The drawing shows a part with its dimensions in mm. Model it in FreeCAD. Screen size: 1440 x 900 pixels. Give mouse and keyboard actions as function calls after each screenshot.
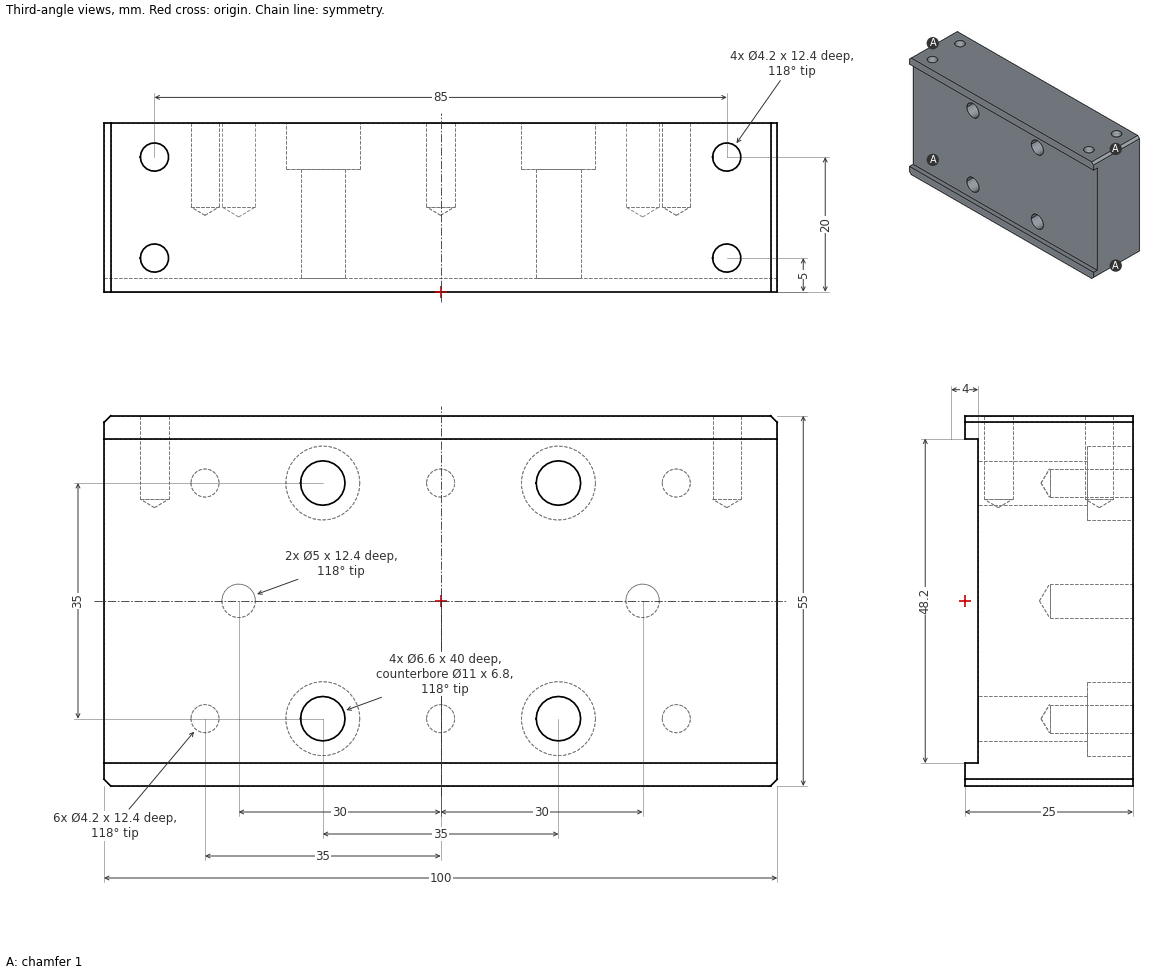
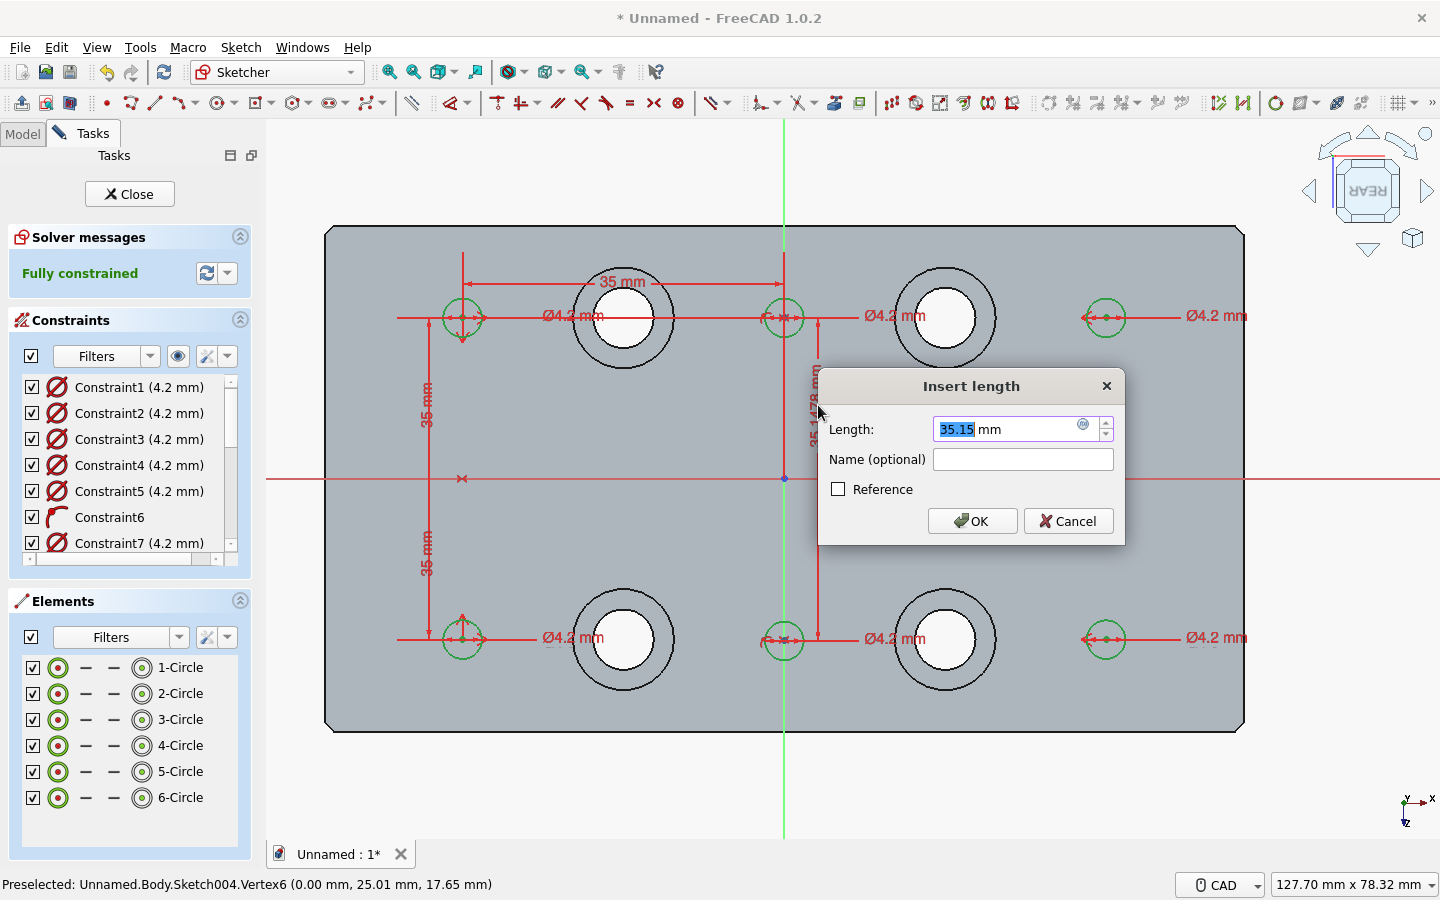
text(35)
key(Return)
key(Escape)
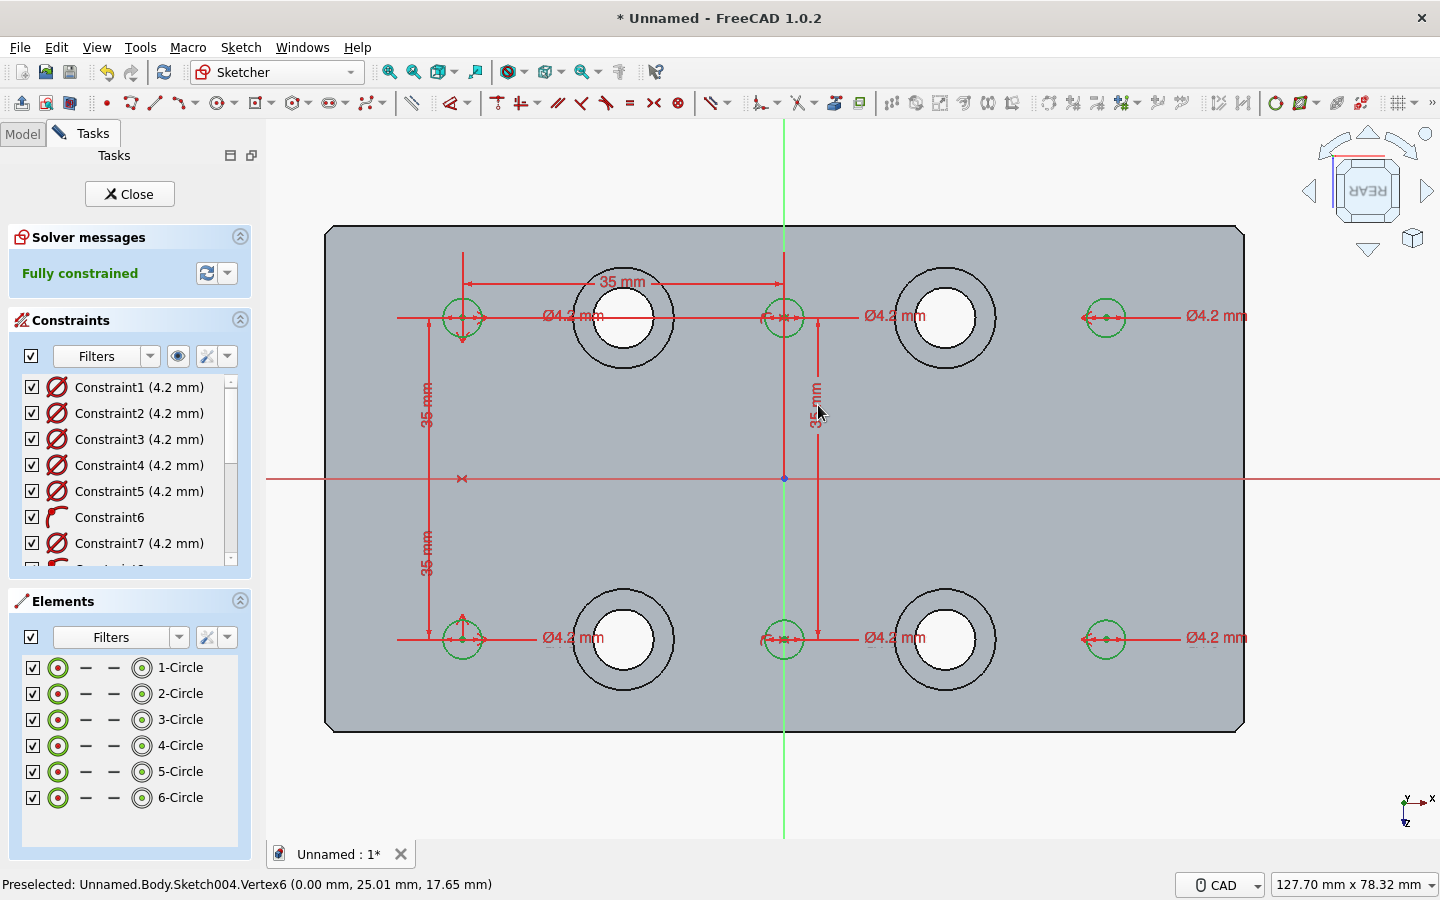
click(130, 194)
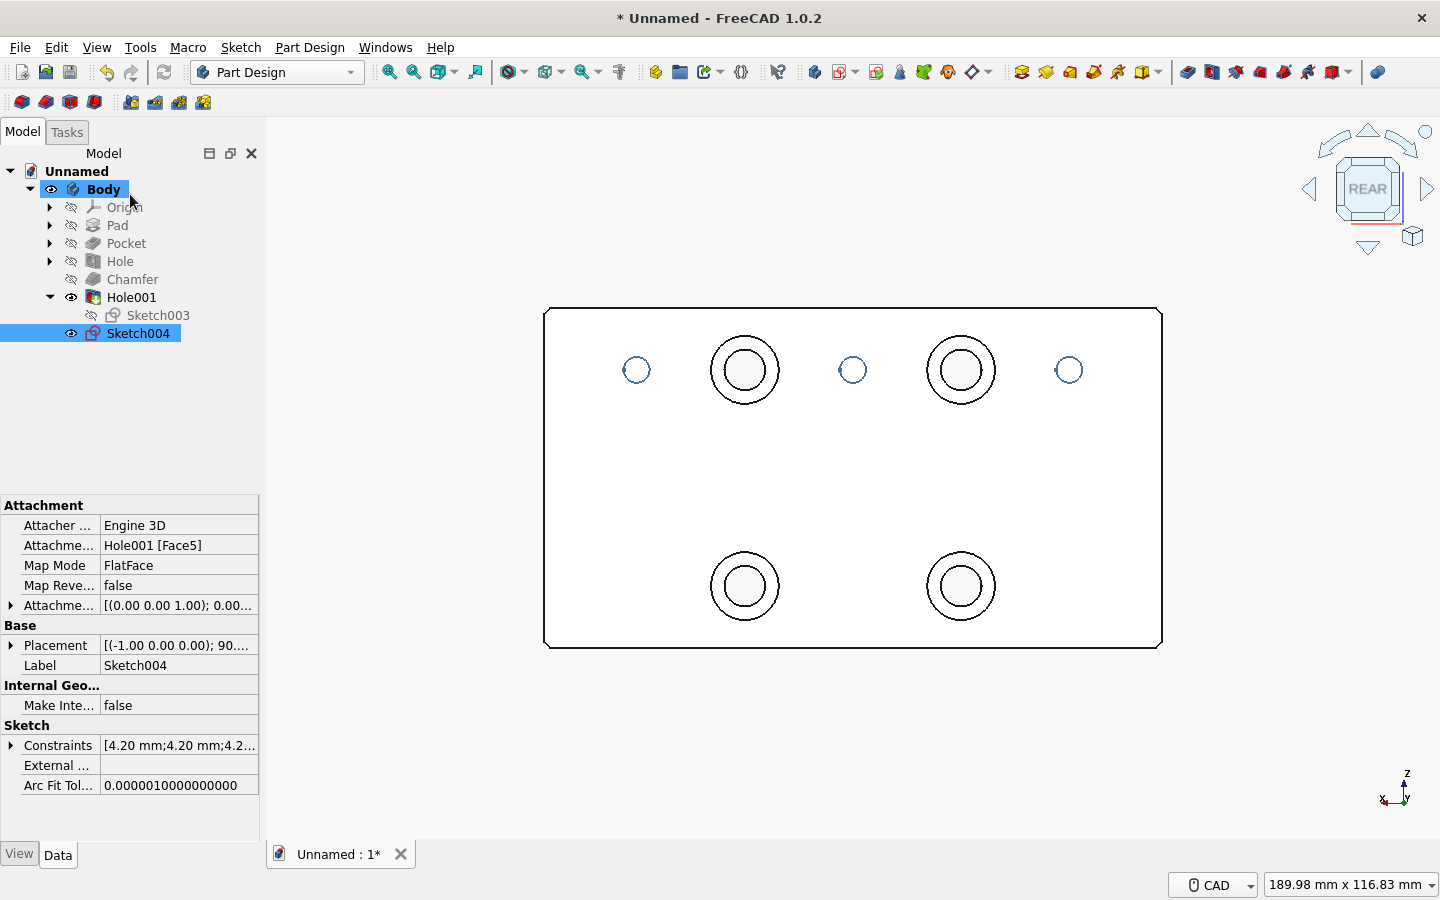
click(1212, 72)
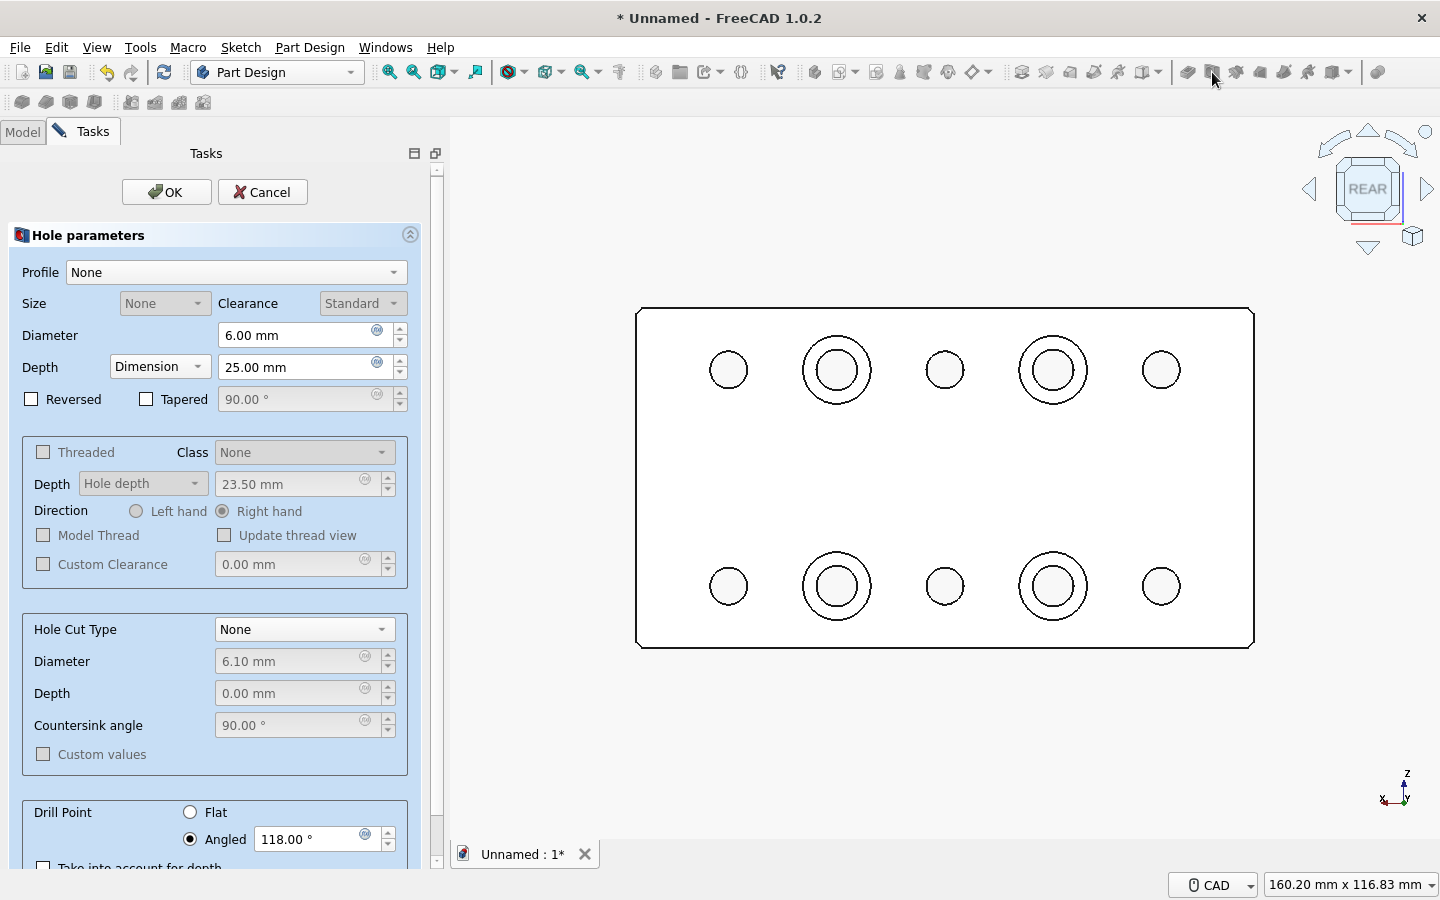
triple_click(305, 335)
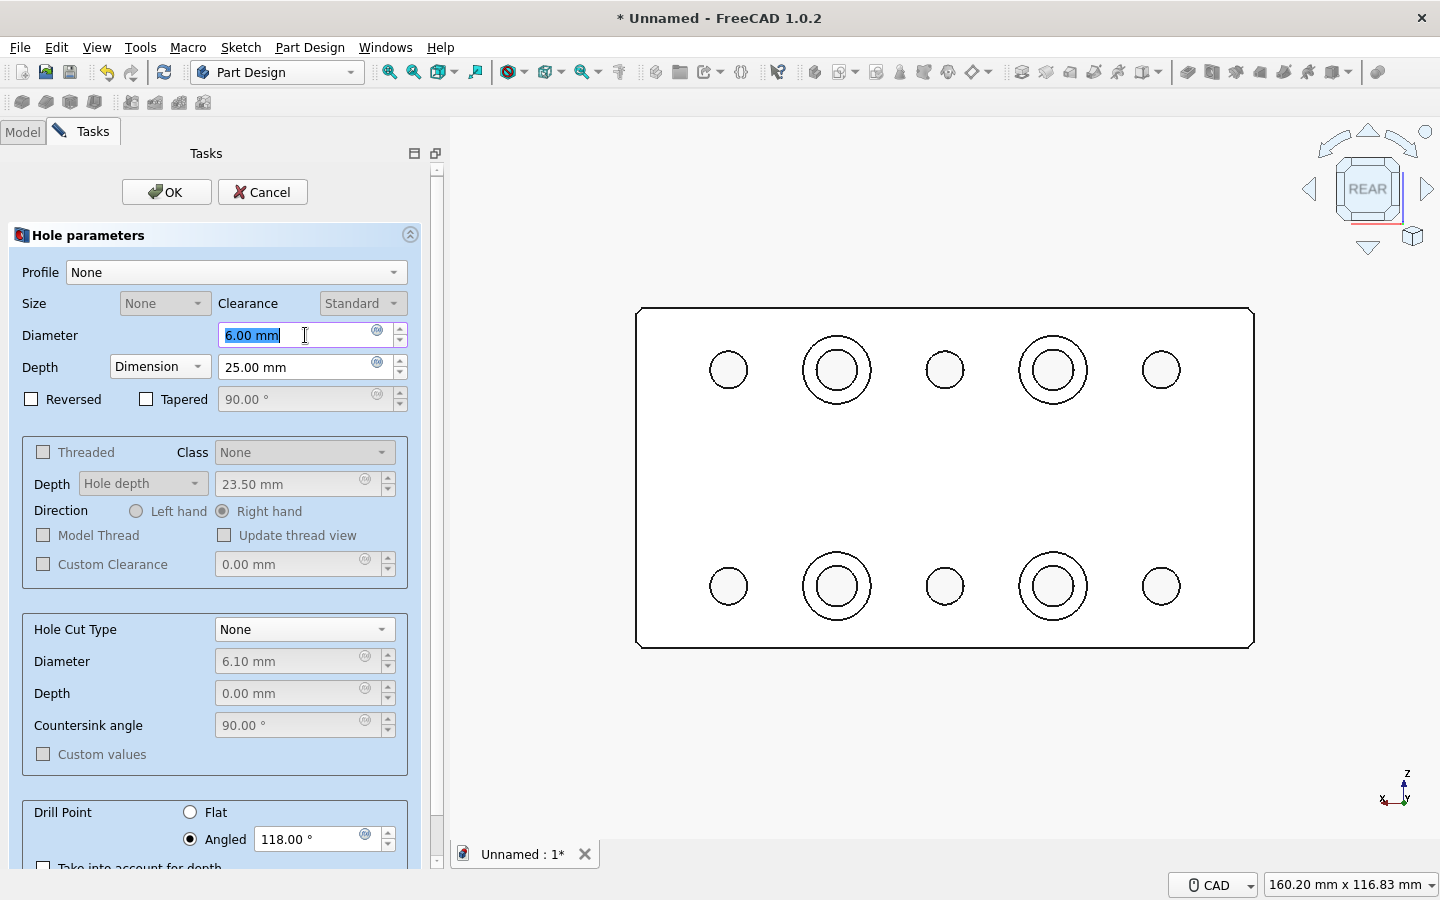
text(4.2)
key(Tab)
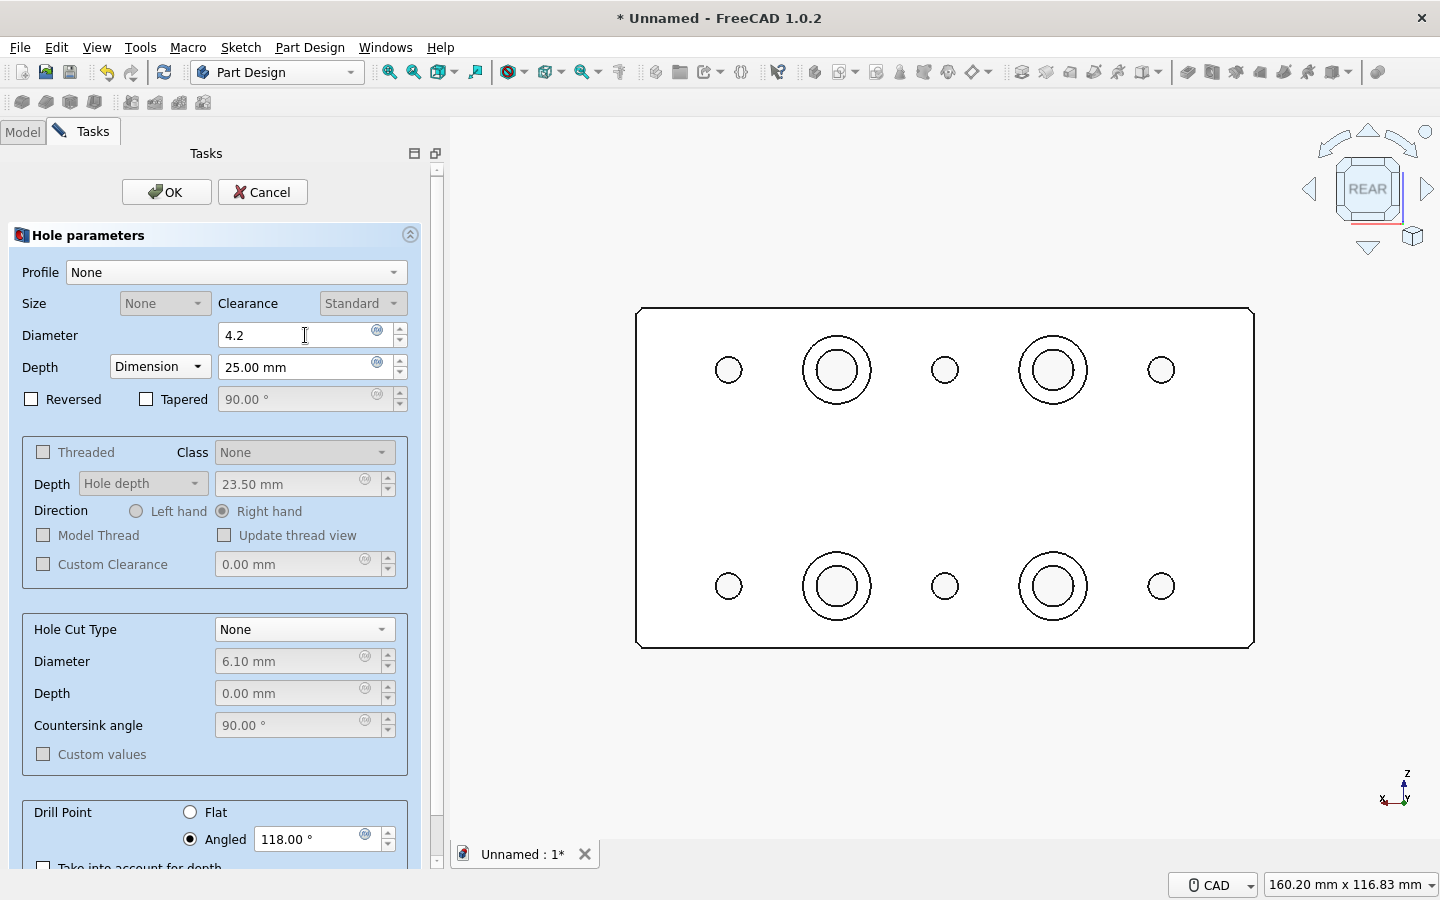
triple_click(305, 367)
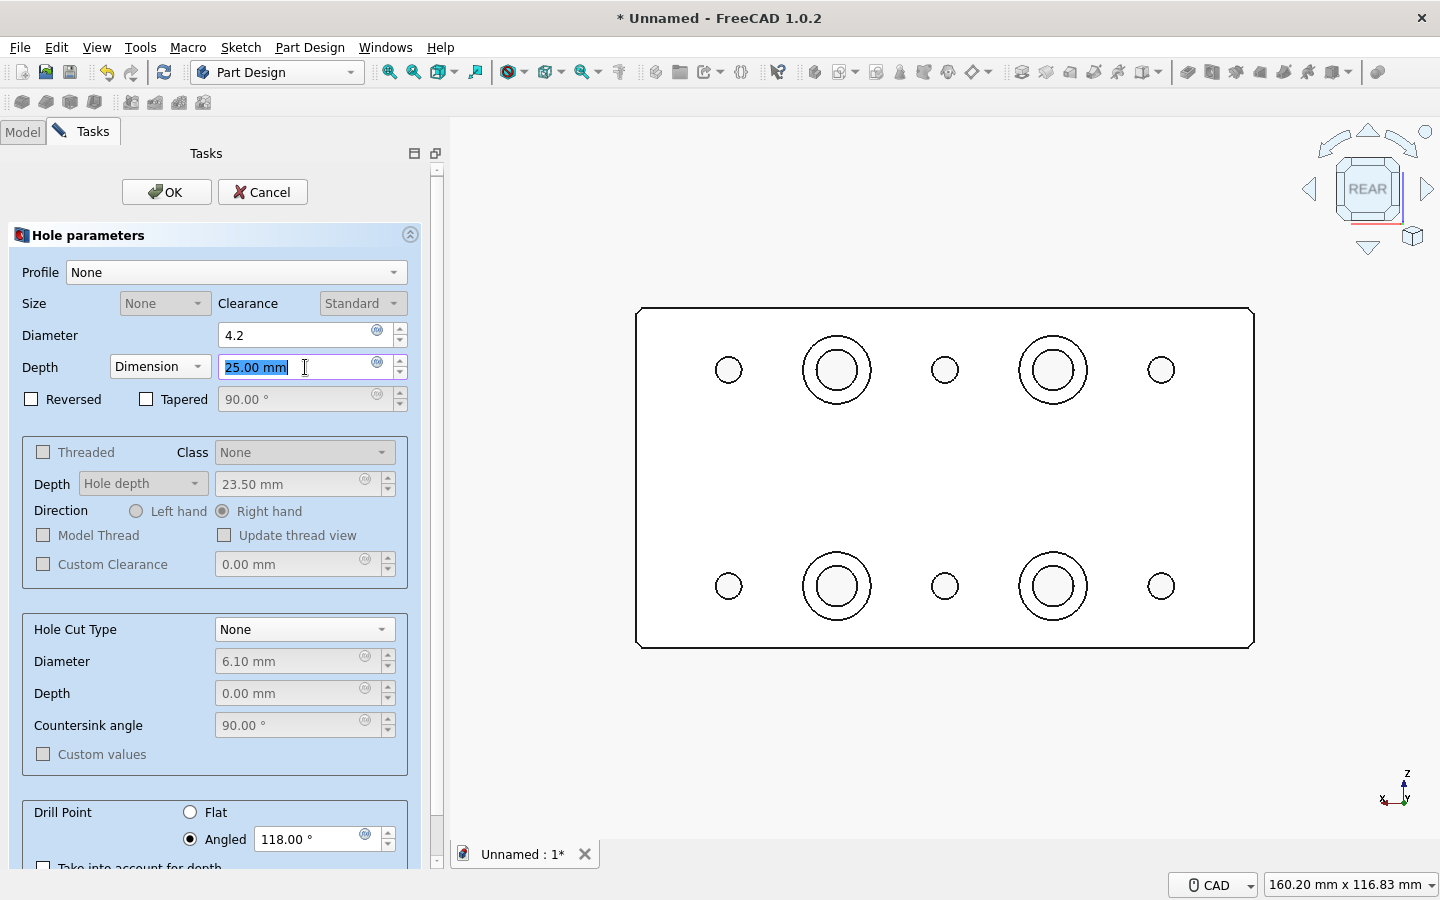
text(12.4)
key(Tab)